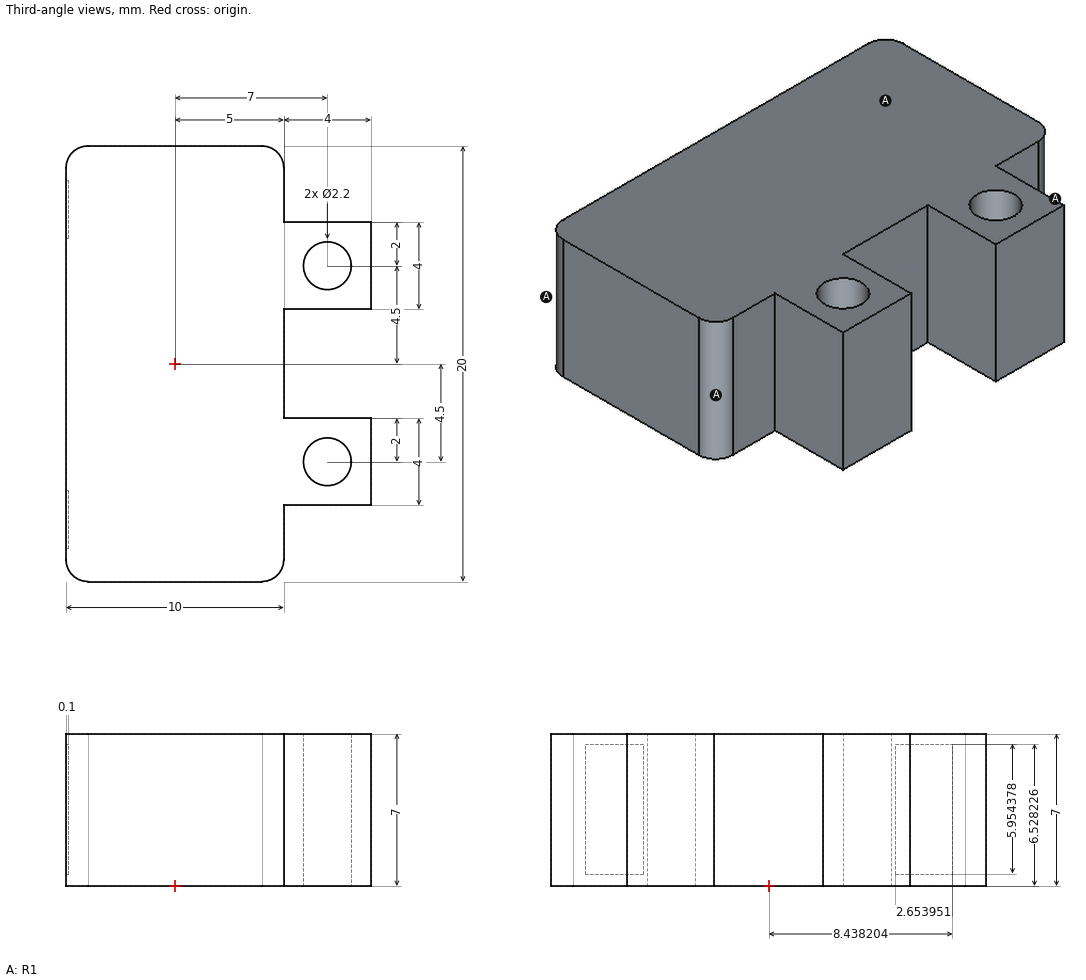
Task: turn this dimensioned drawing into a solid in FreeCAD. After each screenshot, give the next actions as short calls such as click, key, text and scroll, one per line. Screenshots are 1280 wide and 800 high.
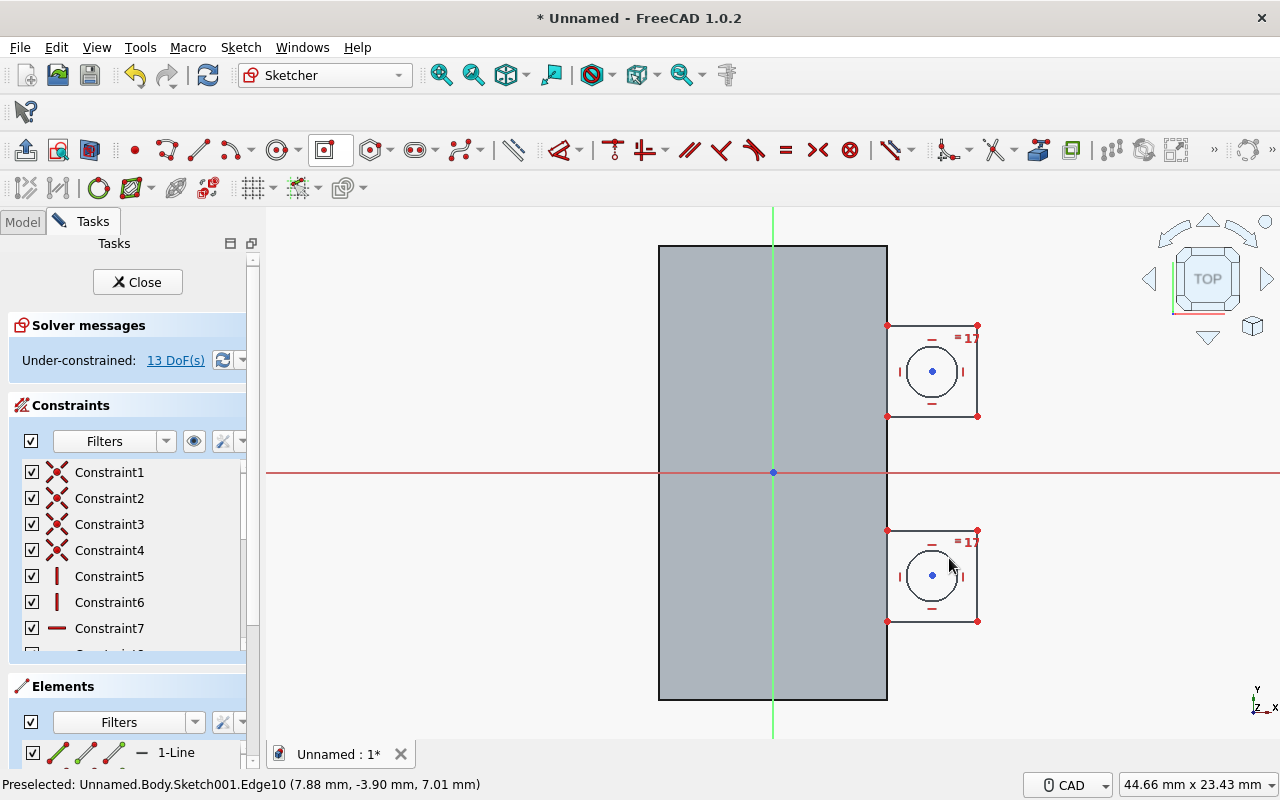
click(950, 354)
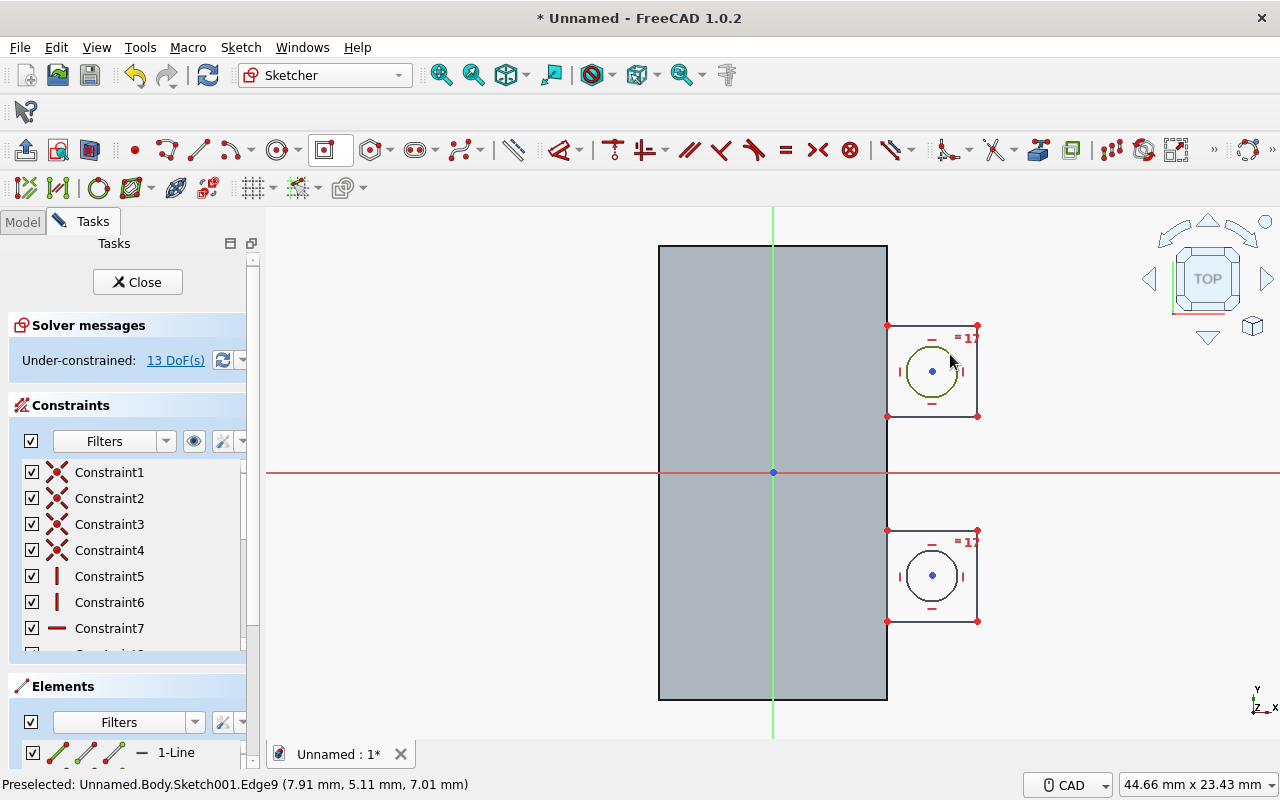
key(k)
key(o)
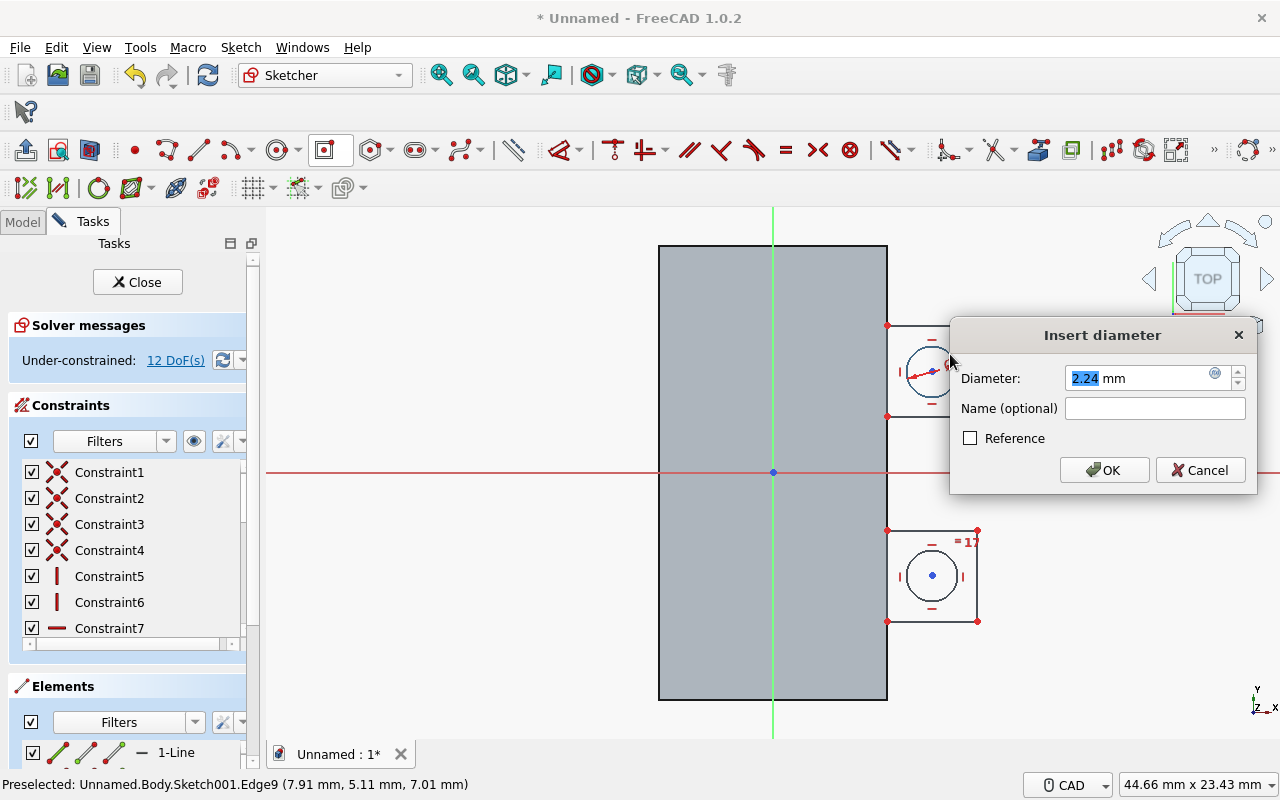
text(2.2)
key(Return)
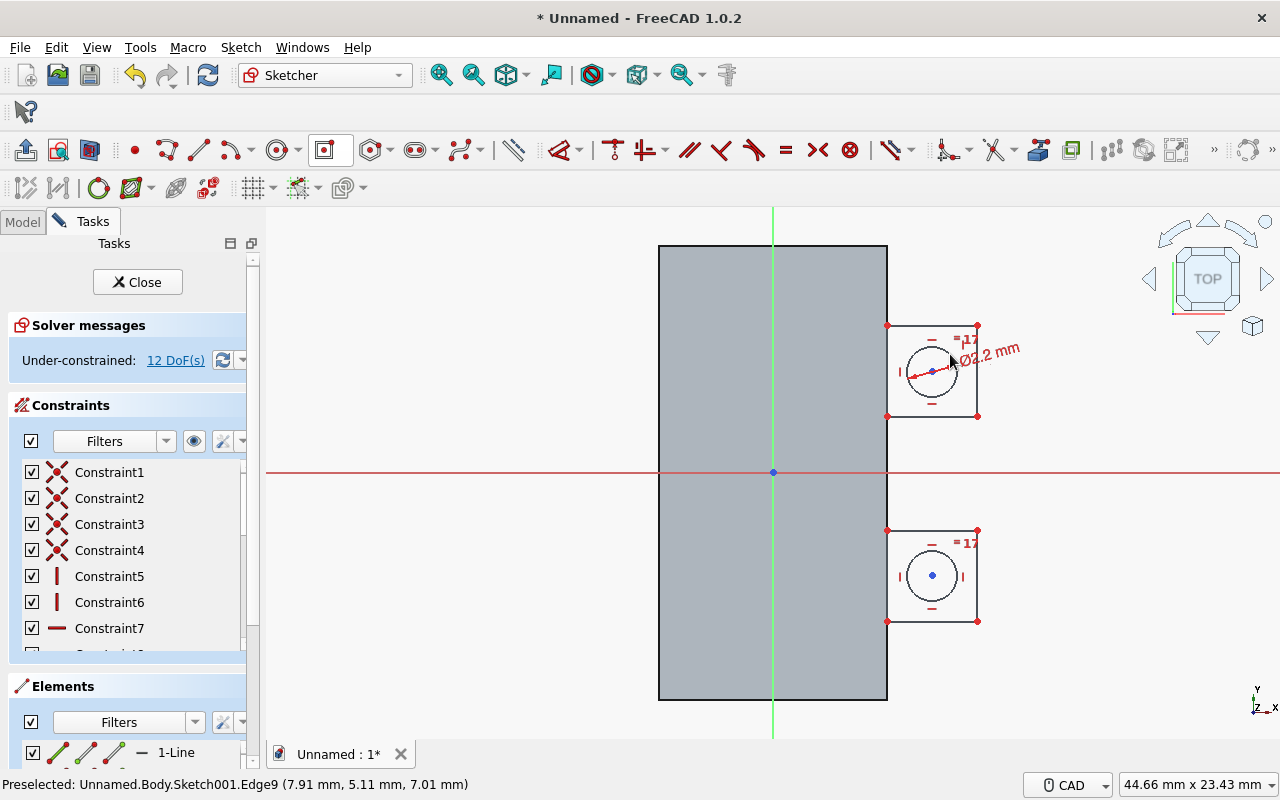
click(887, 353)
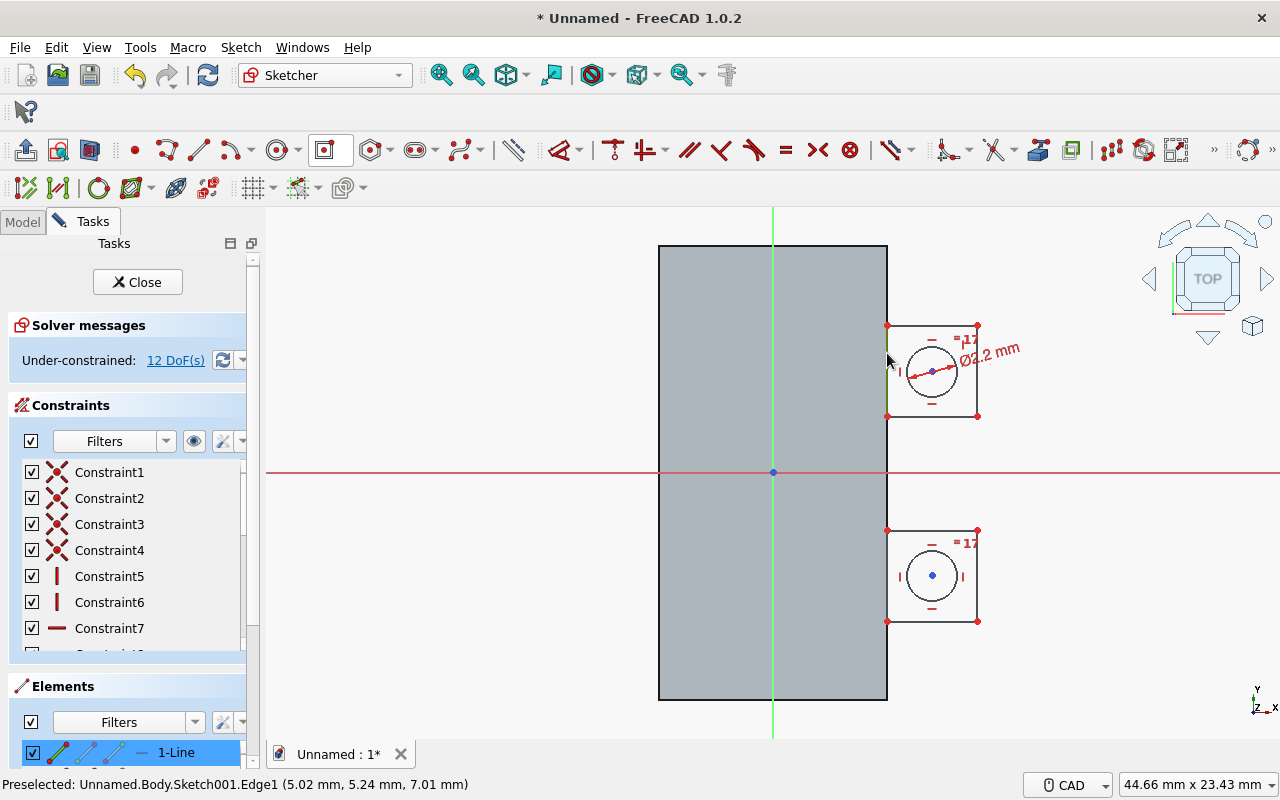
key(i)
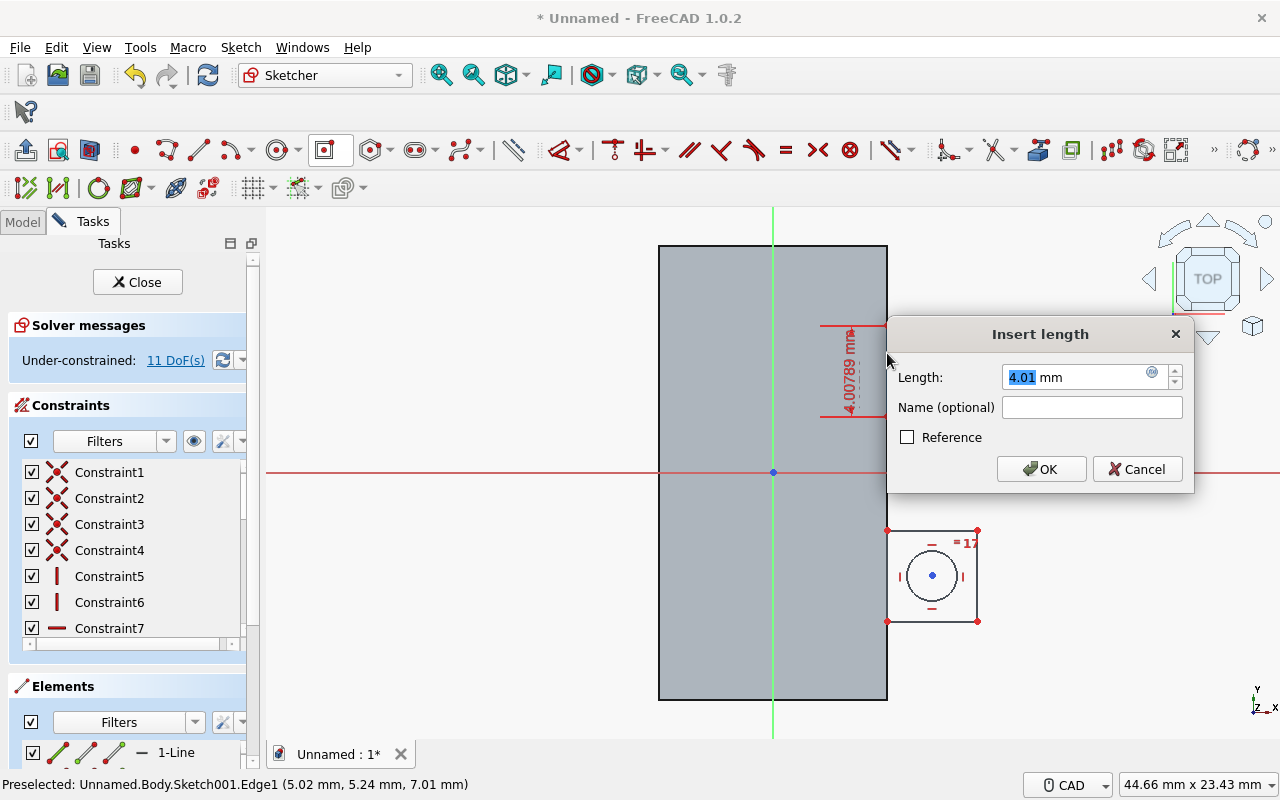
text(4)
key(Return)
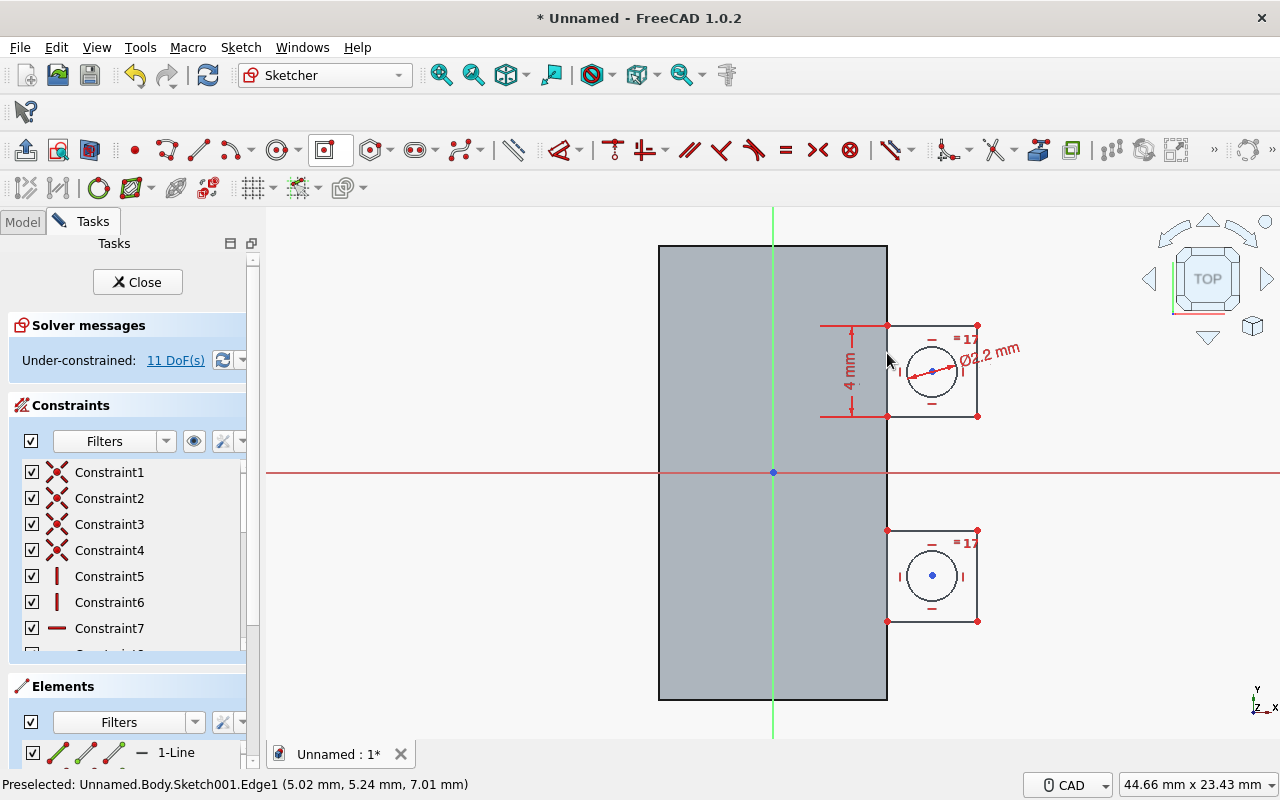
click(914, 417)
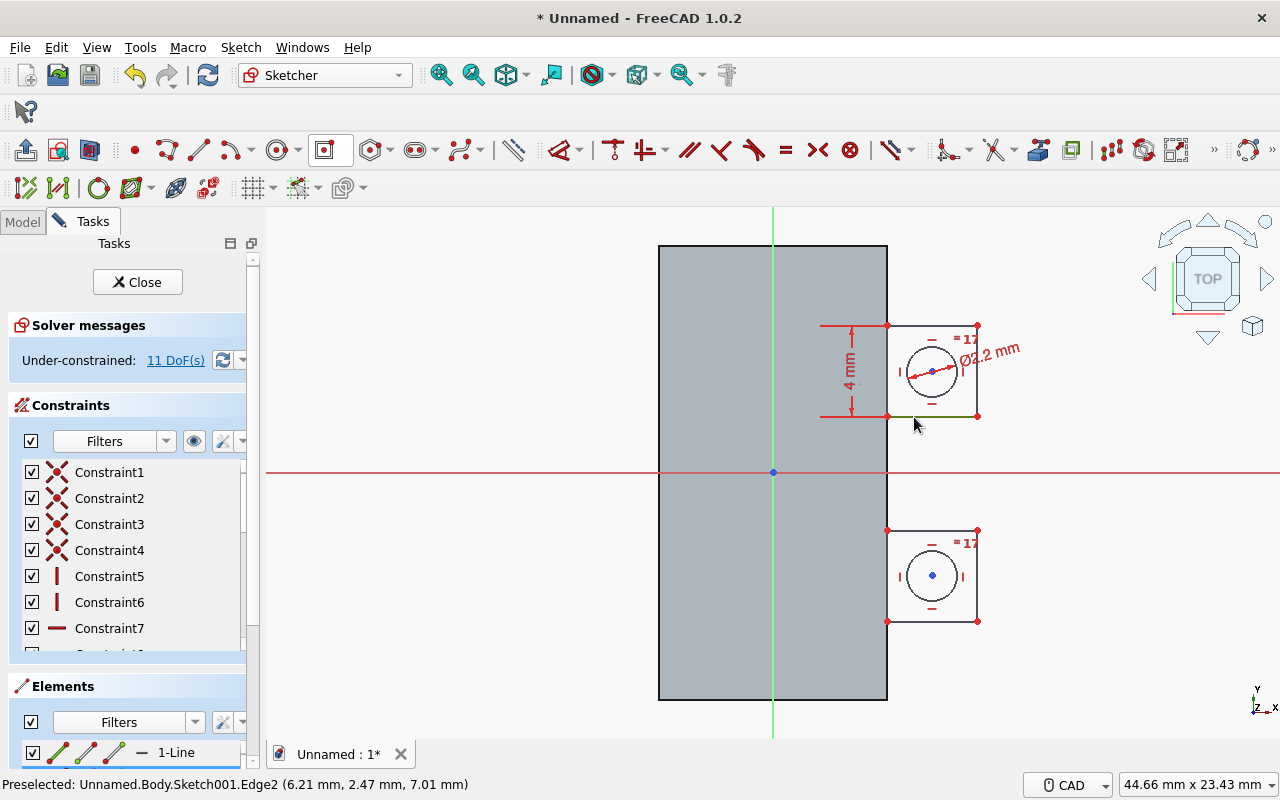
key(l)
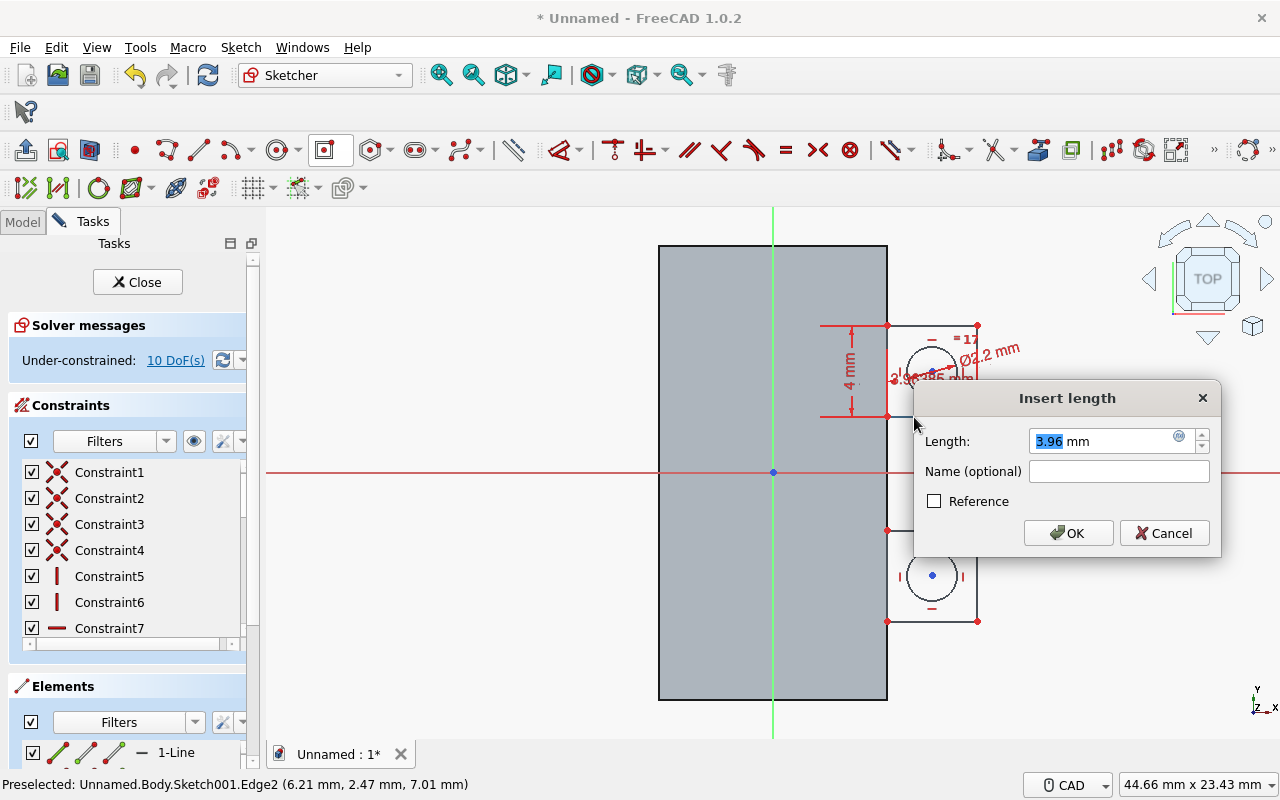
text(4)
key(Return)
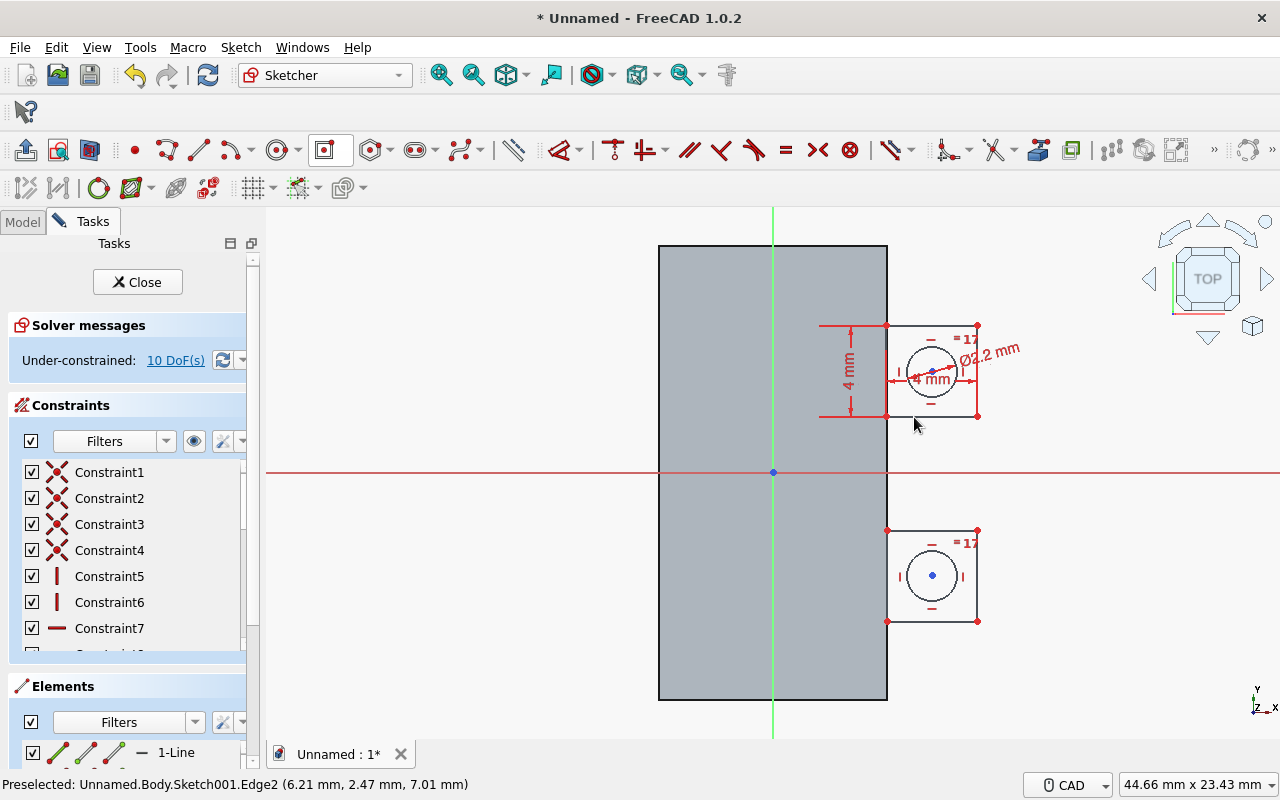
click(887, 558)